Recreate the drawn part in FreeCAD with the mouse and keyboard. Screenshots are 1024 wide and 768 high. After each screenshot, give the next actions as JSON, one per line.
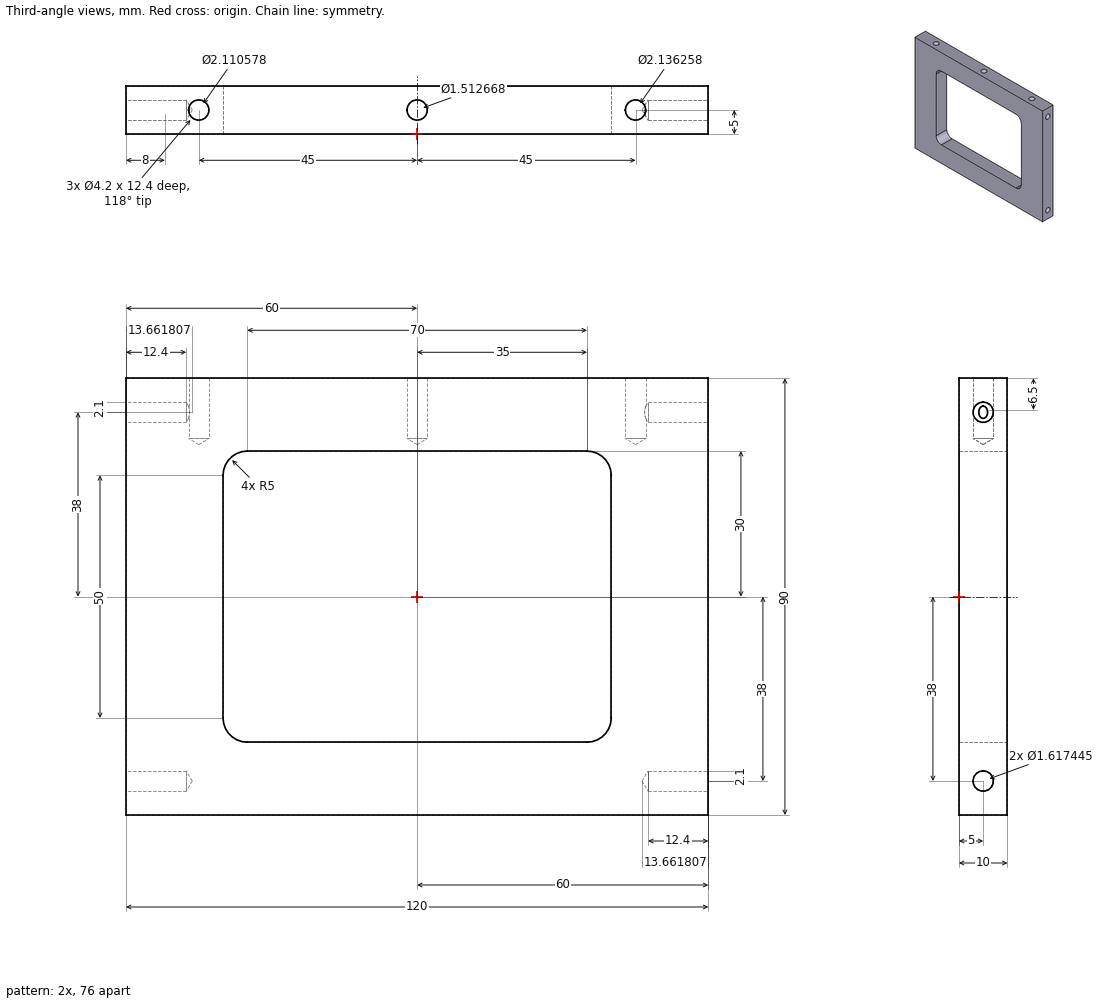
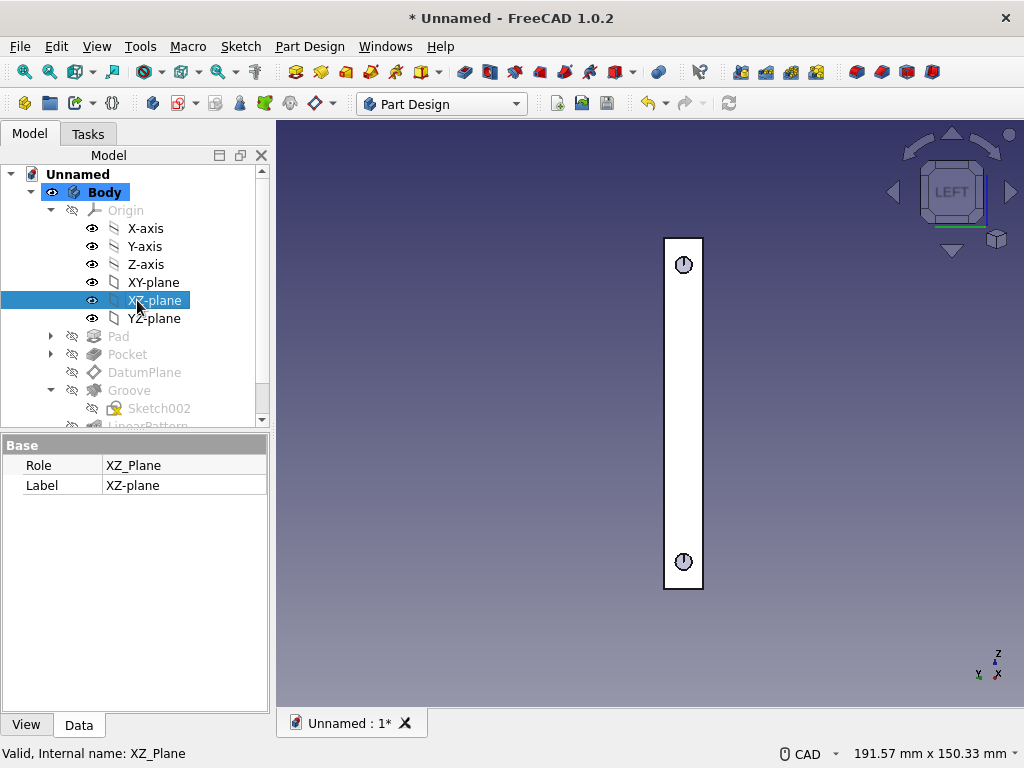
{"action": "left_click", "coordinate": [314, 104]}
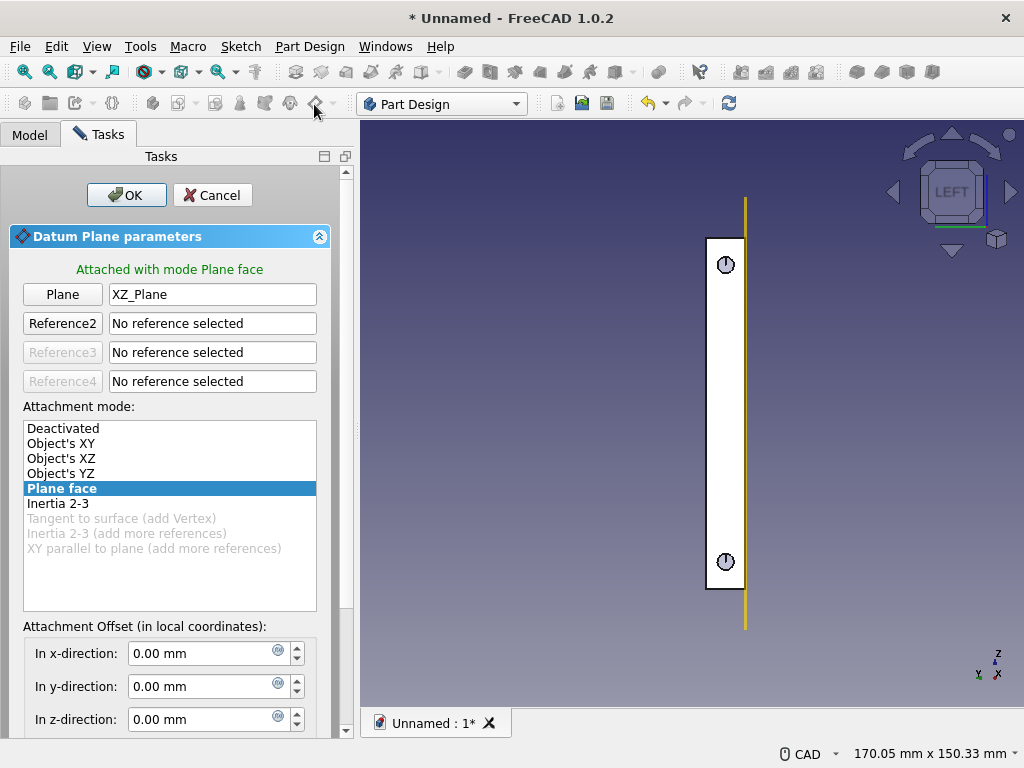
{"action": "triple_click", "coordinate": [210, 720]}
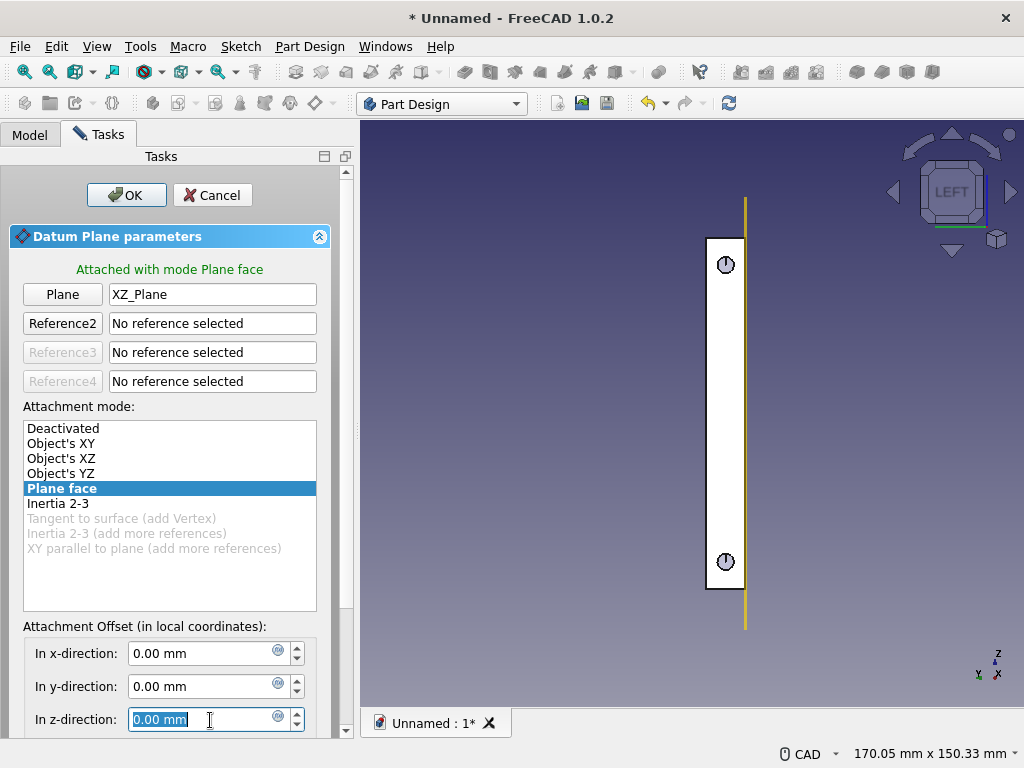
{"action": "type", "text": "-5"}
{"action": "key", "text": "Tab"}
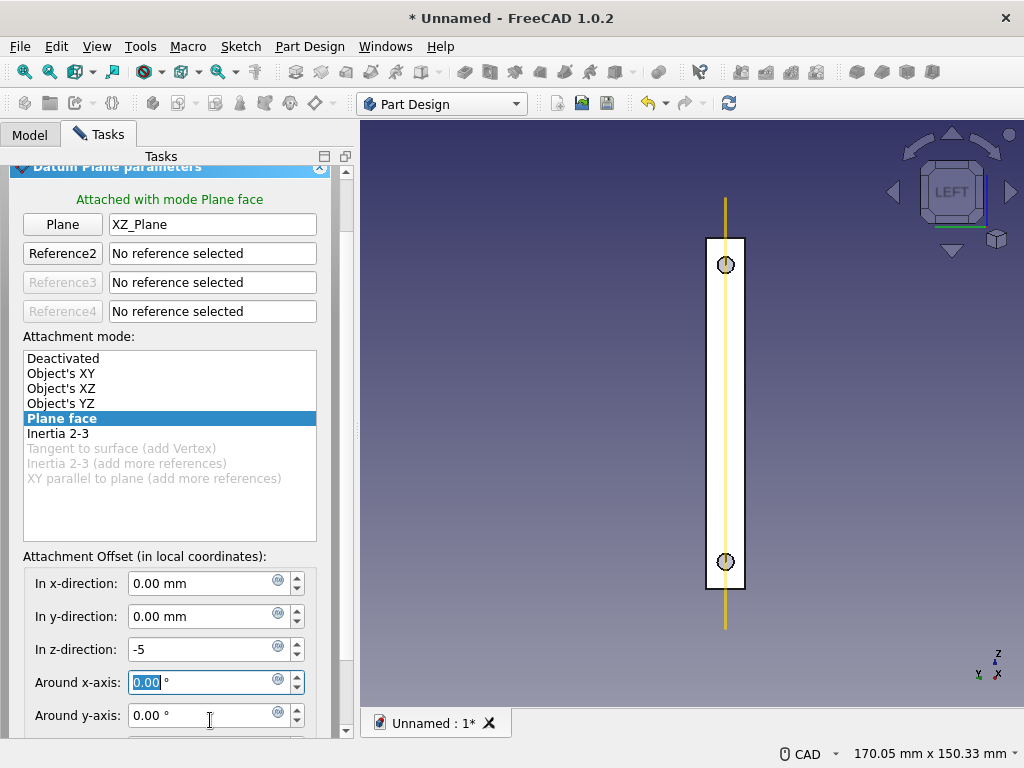
{"action": "scroll", "coordinate": [346, 452], "scroll_direction": "up", "scroll_amount": 2}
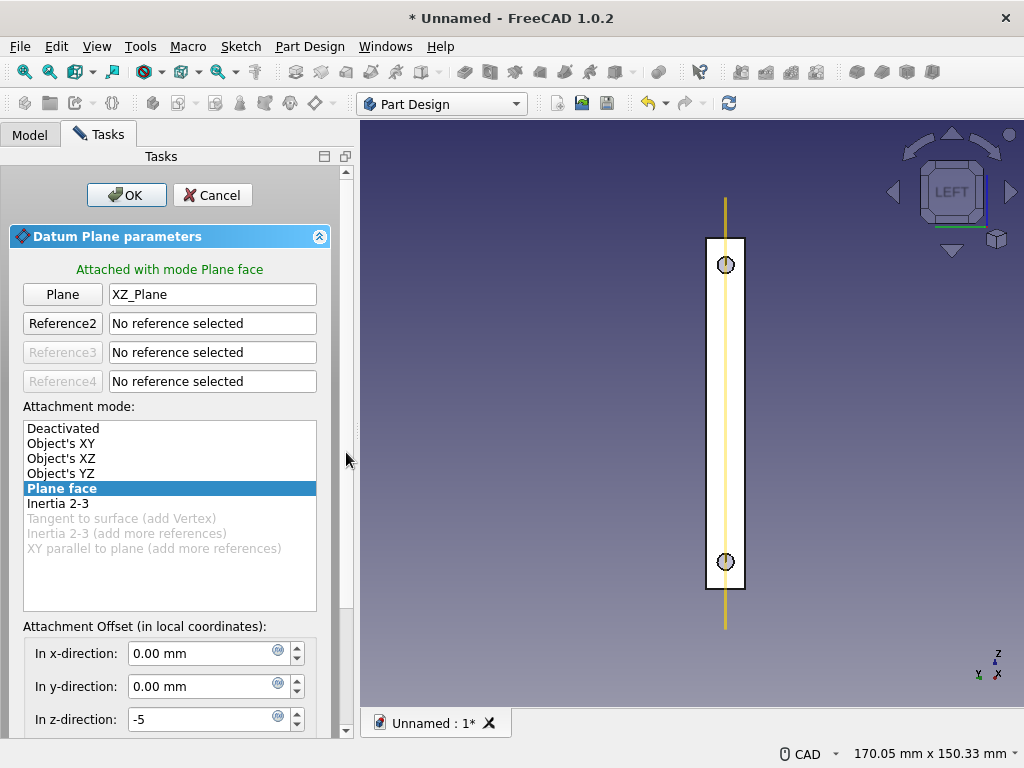
{"action": "left_click", "coordinate": [127, 195]}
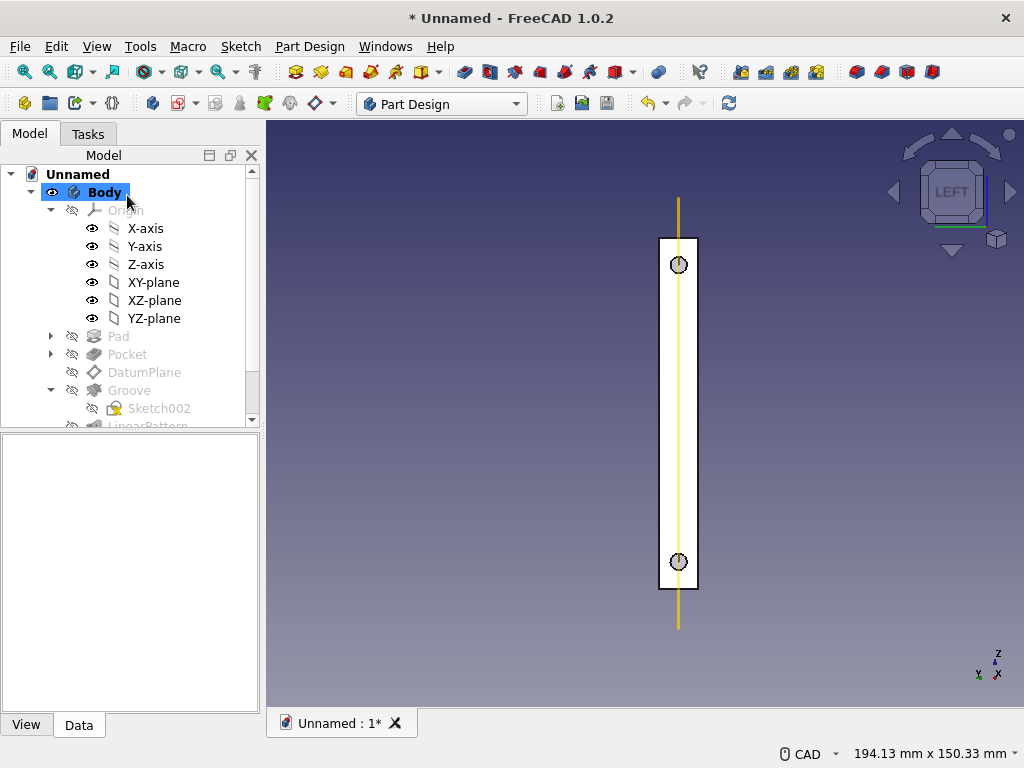
{"action": "scroll", "coordinate": [101, 296], "scroll_direction": "down", "scroll_amount": 3}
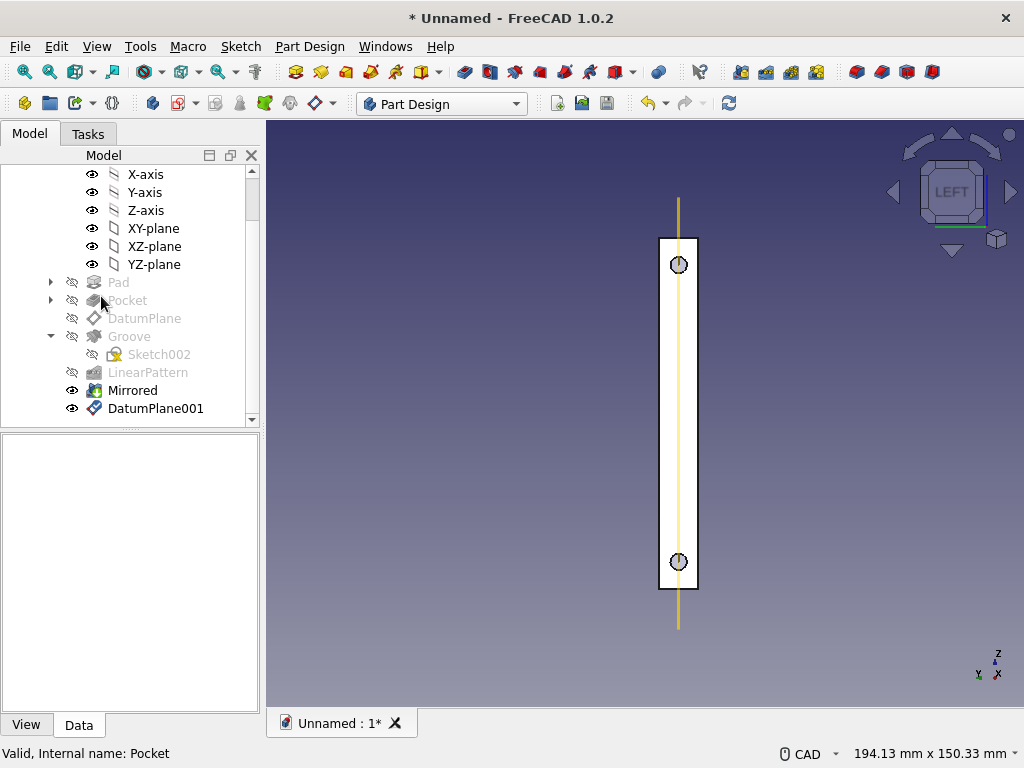
{"action": "left_click", "coordinate": [117, 408]}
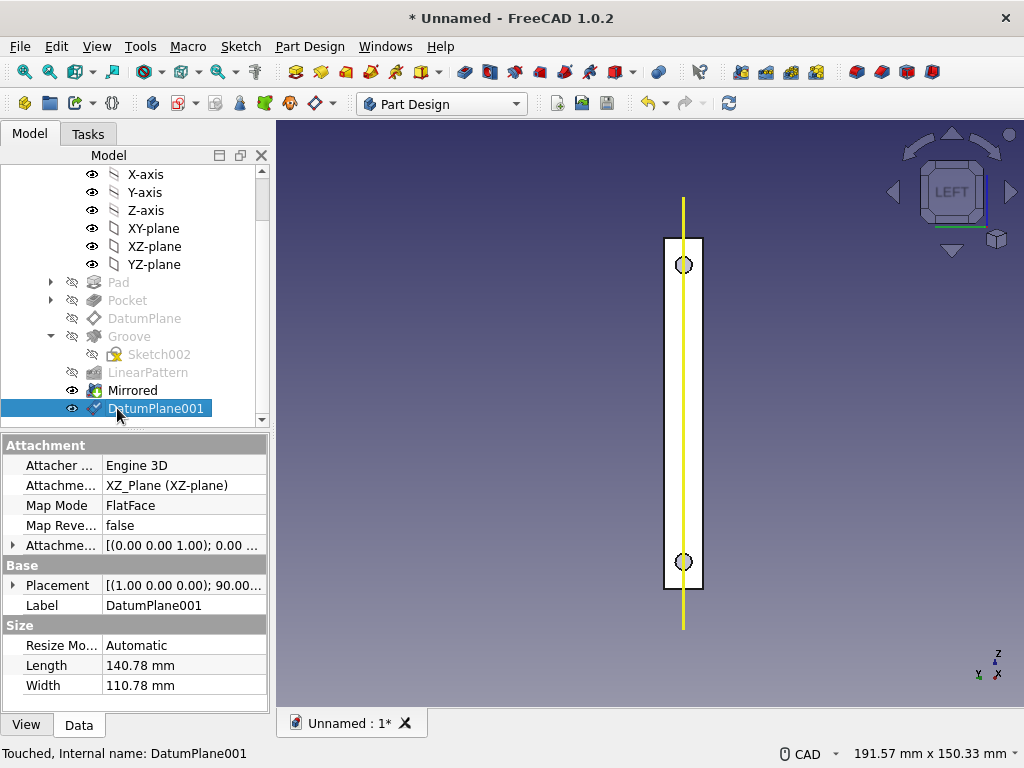
{"action": "left_click", "coordinate": [178, 104]}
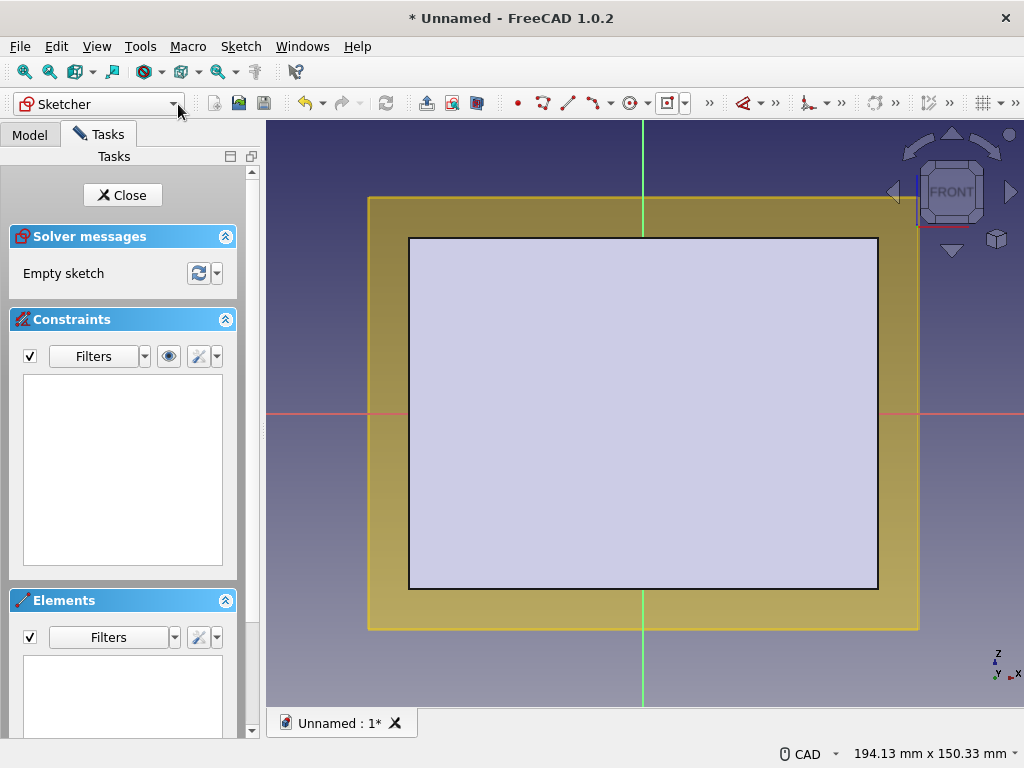
{"action": "left_click", "coordinate": [477, 104]}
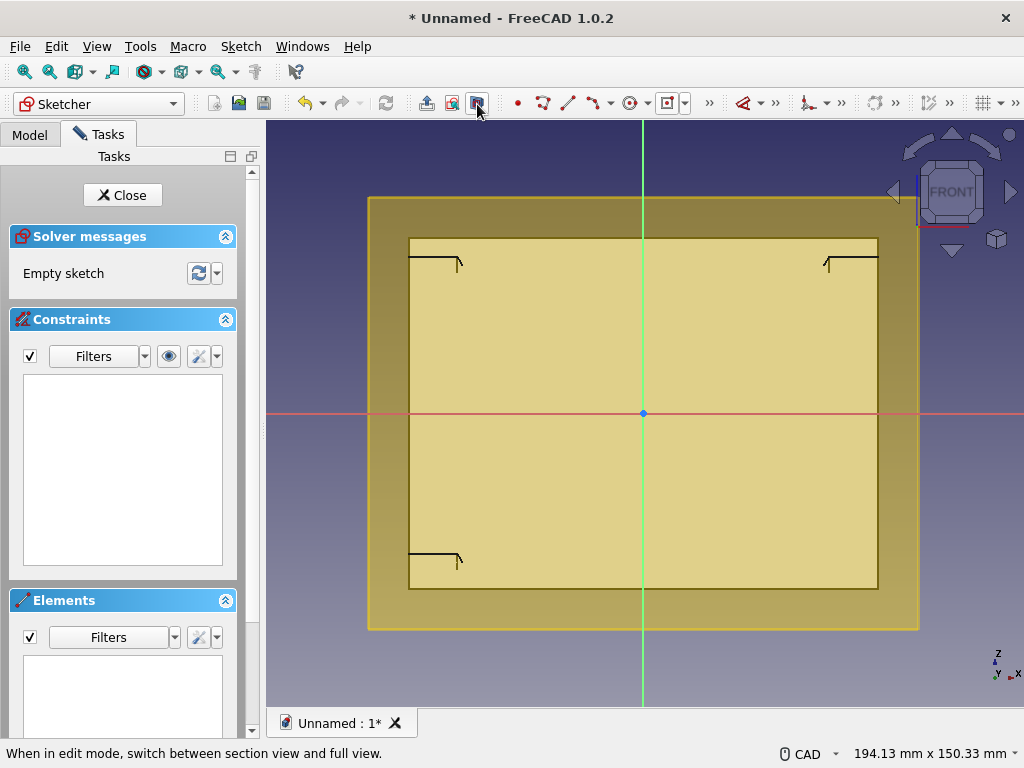
{"action": "scroll", "coordinate": [576, 414], "scroll_direction": "down", "scroll_amount": 5}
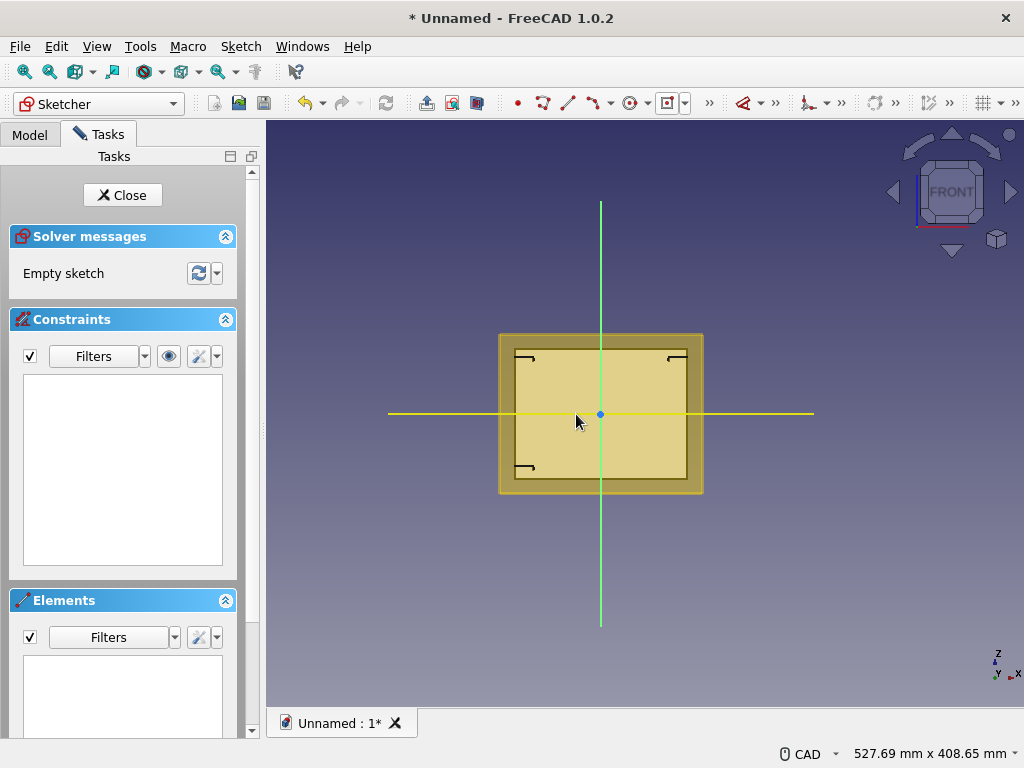
{"action": "scroll", "coordinate": [690, 472], "scroll_direction": "up", "scroll_amount": 13}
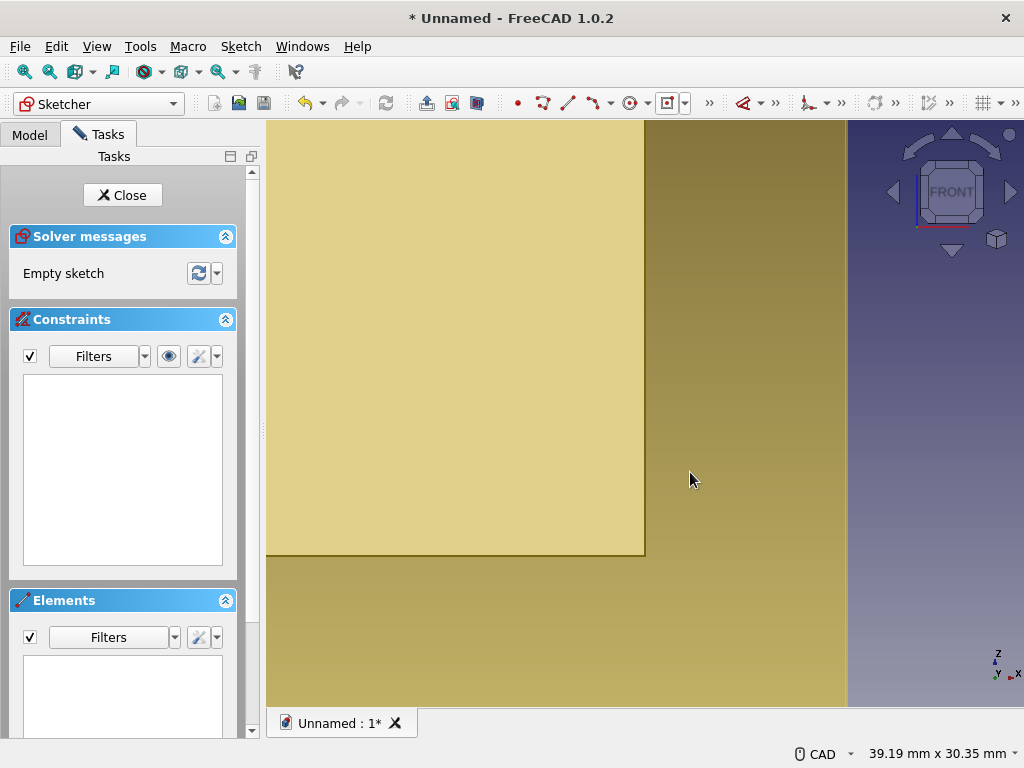
{"action": "left_click", "coordinate": [543, 104]}